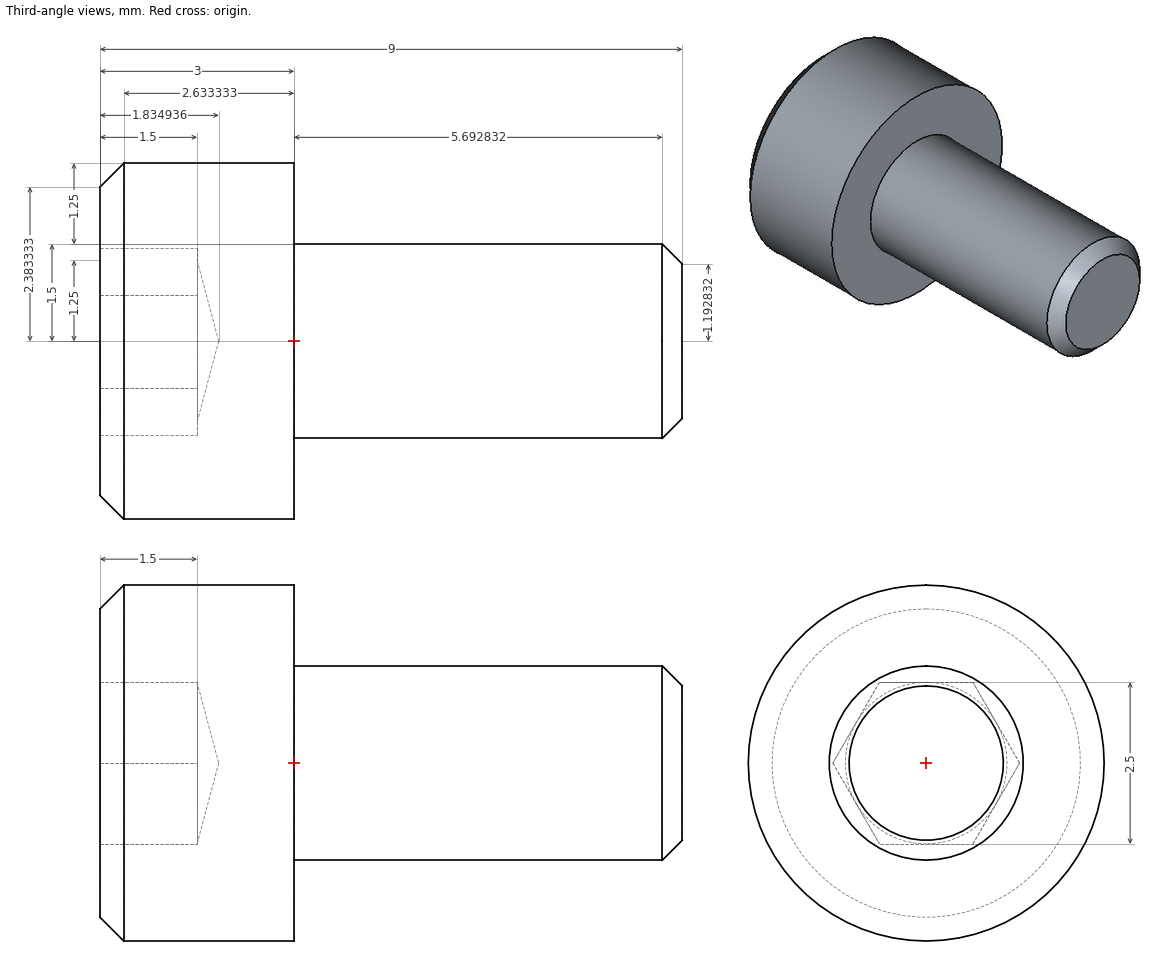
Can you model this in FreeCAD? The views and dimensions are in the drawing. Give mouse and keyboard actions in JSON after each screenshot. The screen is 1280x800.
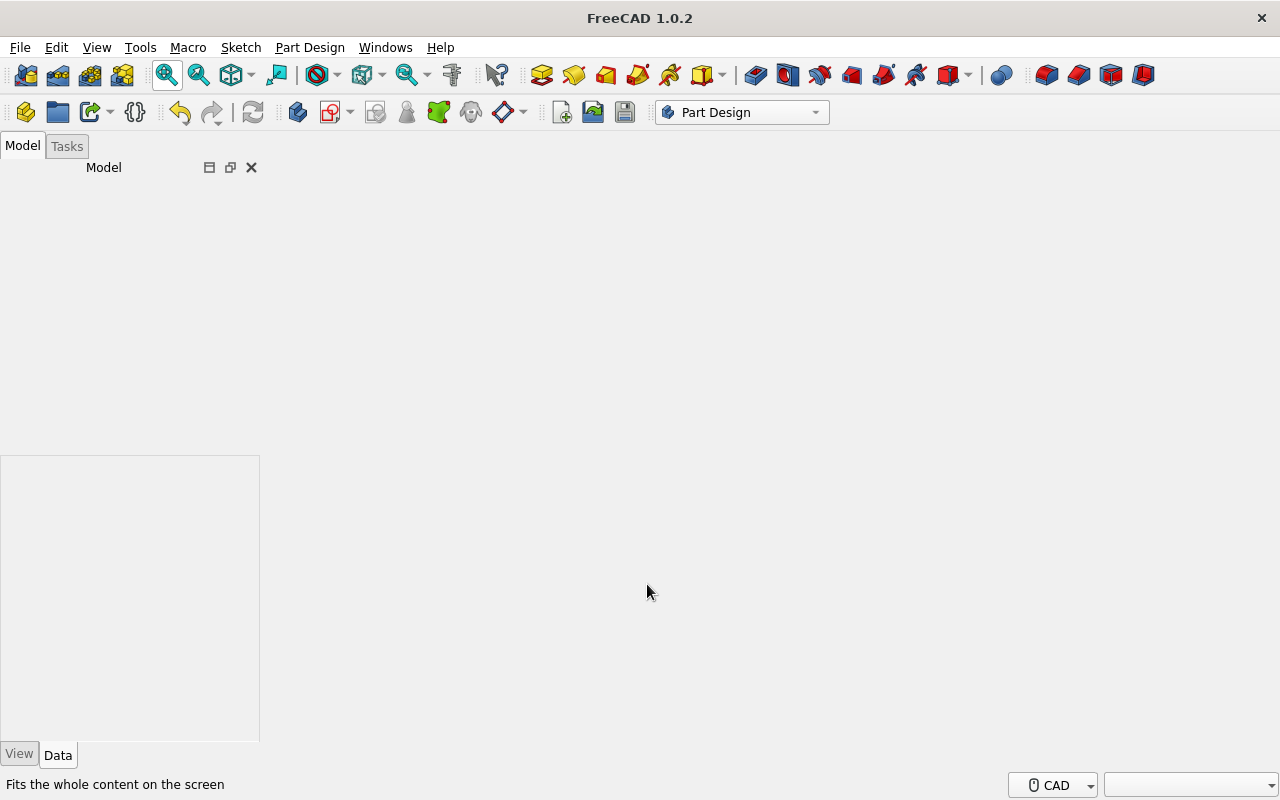
{"action": "left_click", "coordinate": [562, 112]}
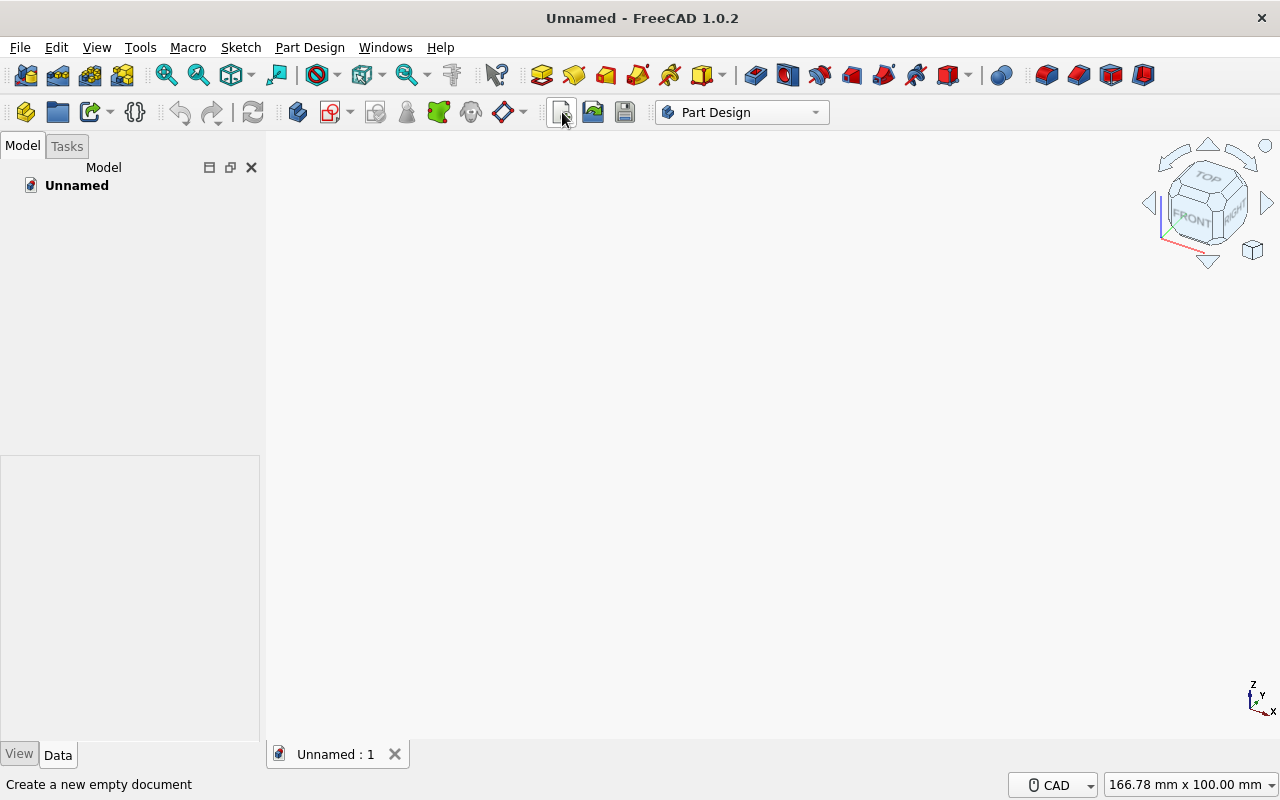
{"action": "left_click", "coordinate": [330, 112]}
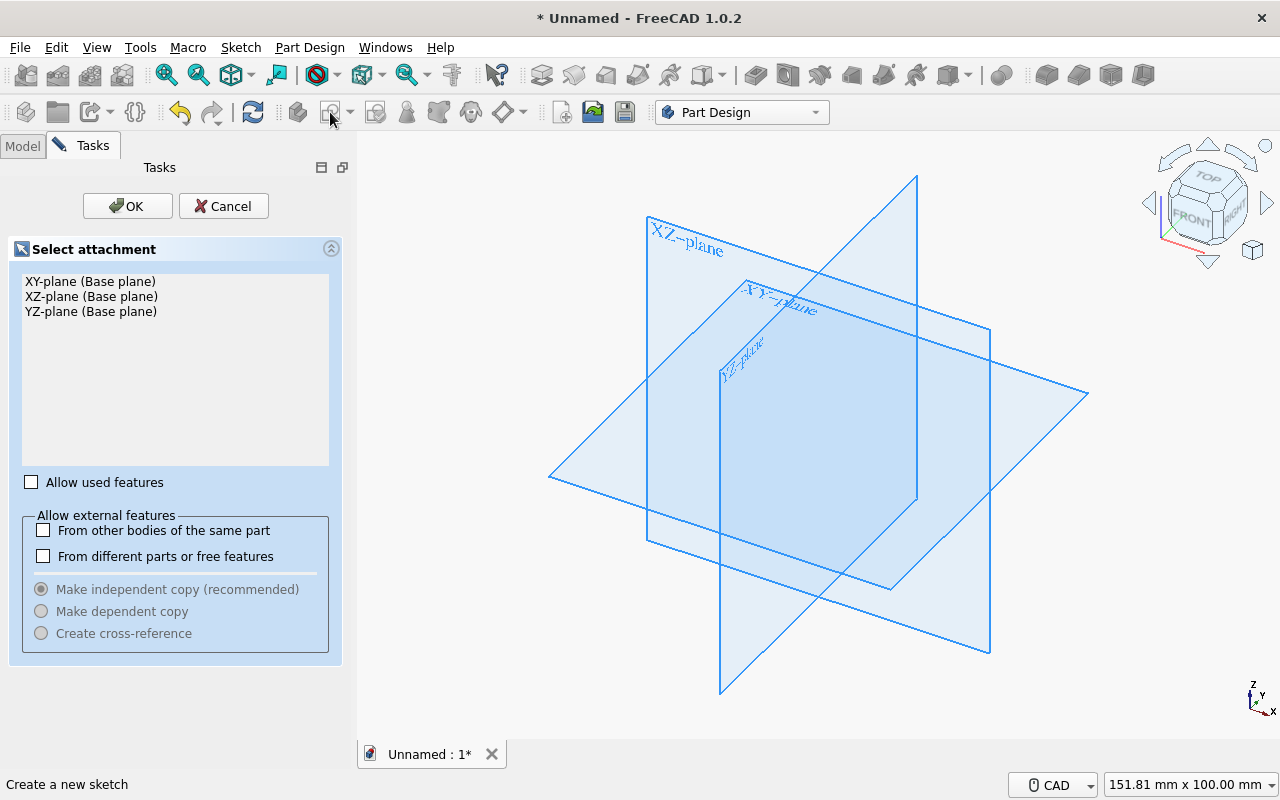
{"action": "left_click", "coordinate": [82, 282]}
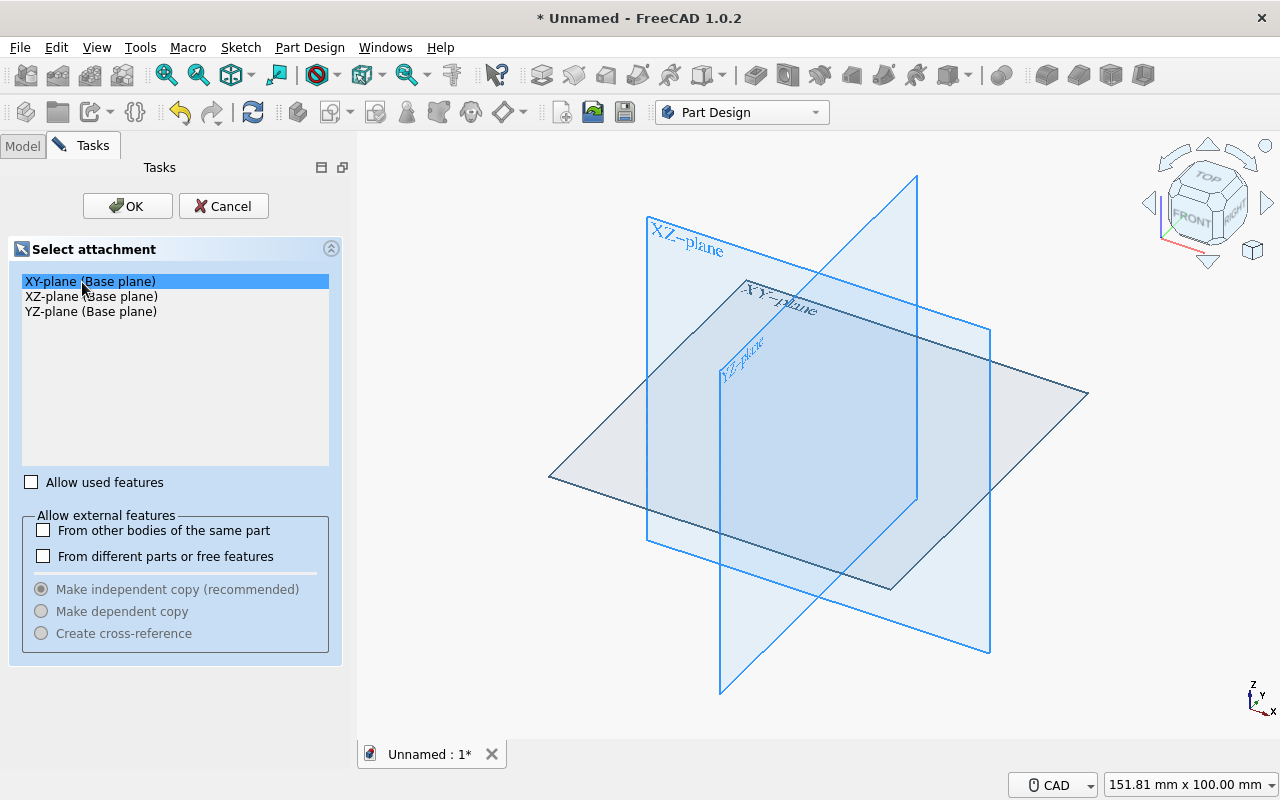
{"action": "left_click", "coordinate": [128, 206]}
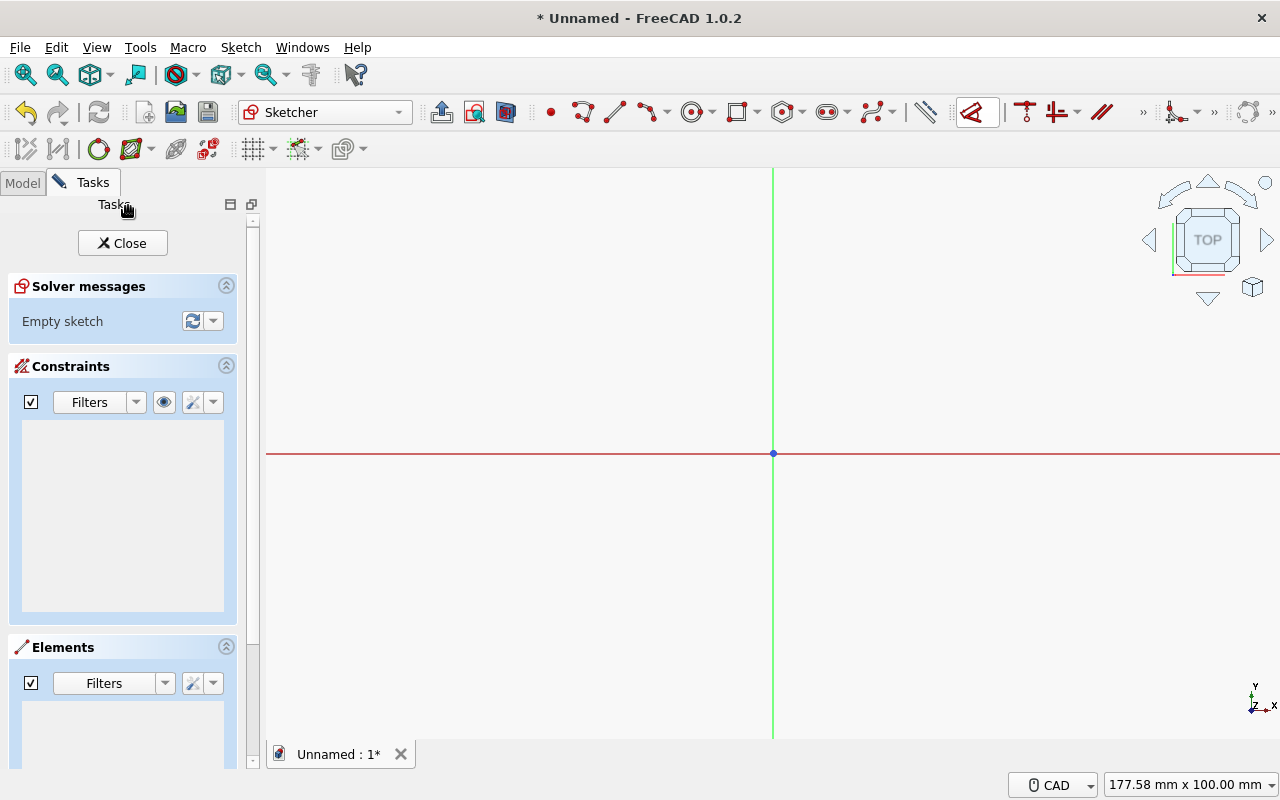
{"action": "scroll", "coordinate": [789, 445], "scroll_direction": "up", "scroll_amount": 12}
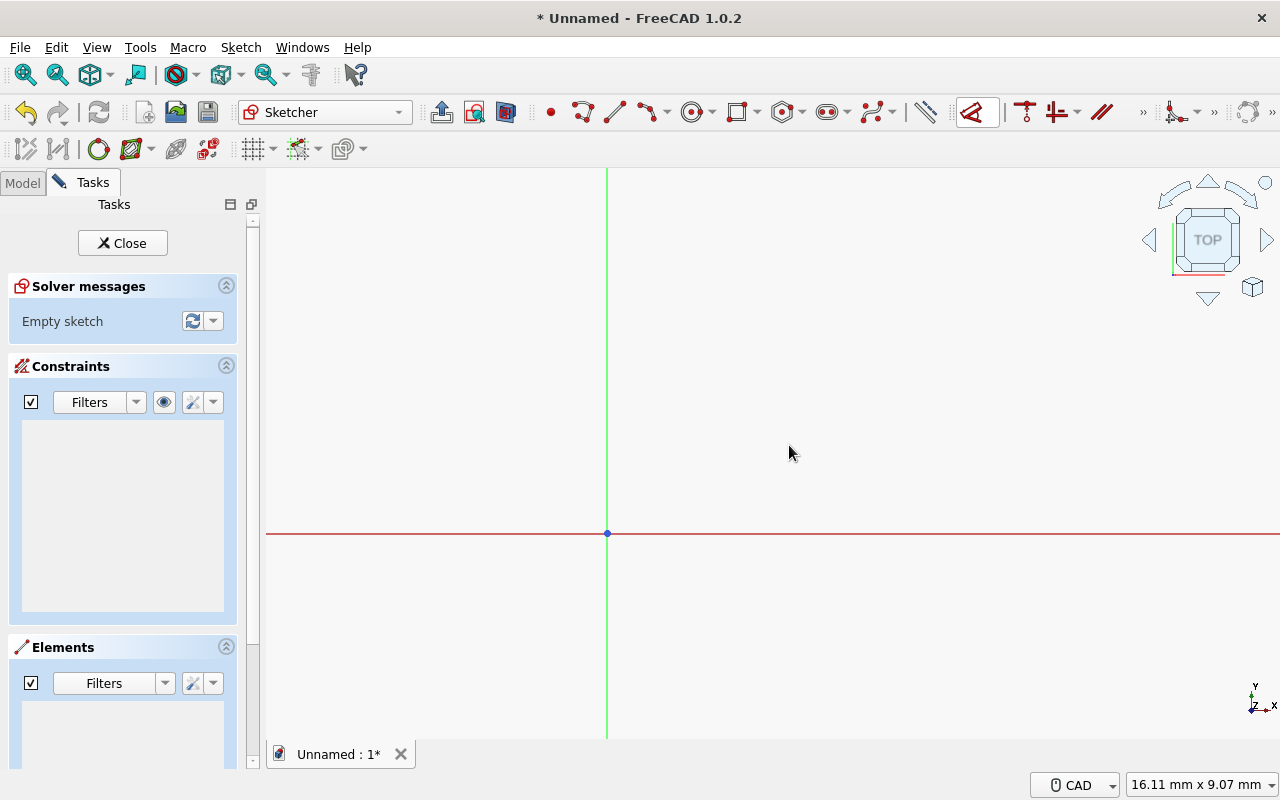
{"action": "left_click", "coordinate": [584, 112]}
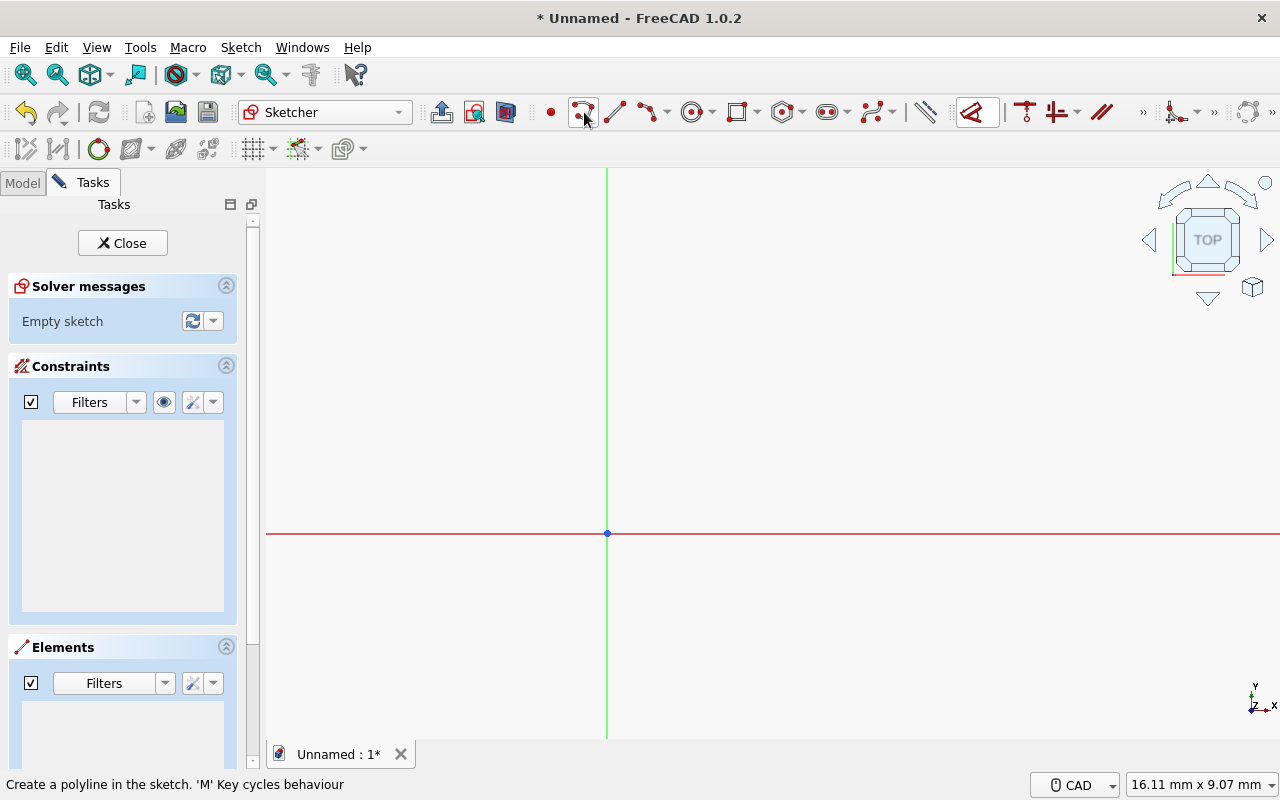
{"action": "left_click", "coordinate": [607, 439]}
{"action": "left_click", "coordinate": [616, 361]}
{"action": "left_click", "coordinate": [442, 361]}
{"action": "left_click", "coordinate": [419, 384]}
{"action": "left_click", "coordinate": [419, 534]}
{"action": "left_click", "coordinate": [985, 525]}
{"action": "left_click", "coordinate": [985, 459]}
{"action": "left_click", "coordinate": [966, 439]}
{"action": "left_click", "coordinate": [607, 440]}
{"action": "key", "text": "Escape"}
{"action": "key", "text": "Escape"}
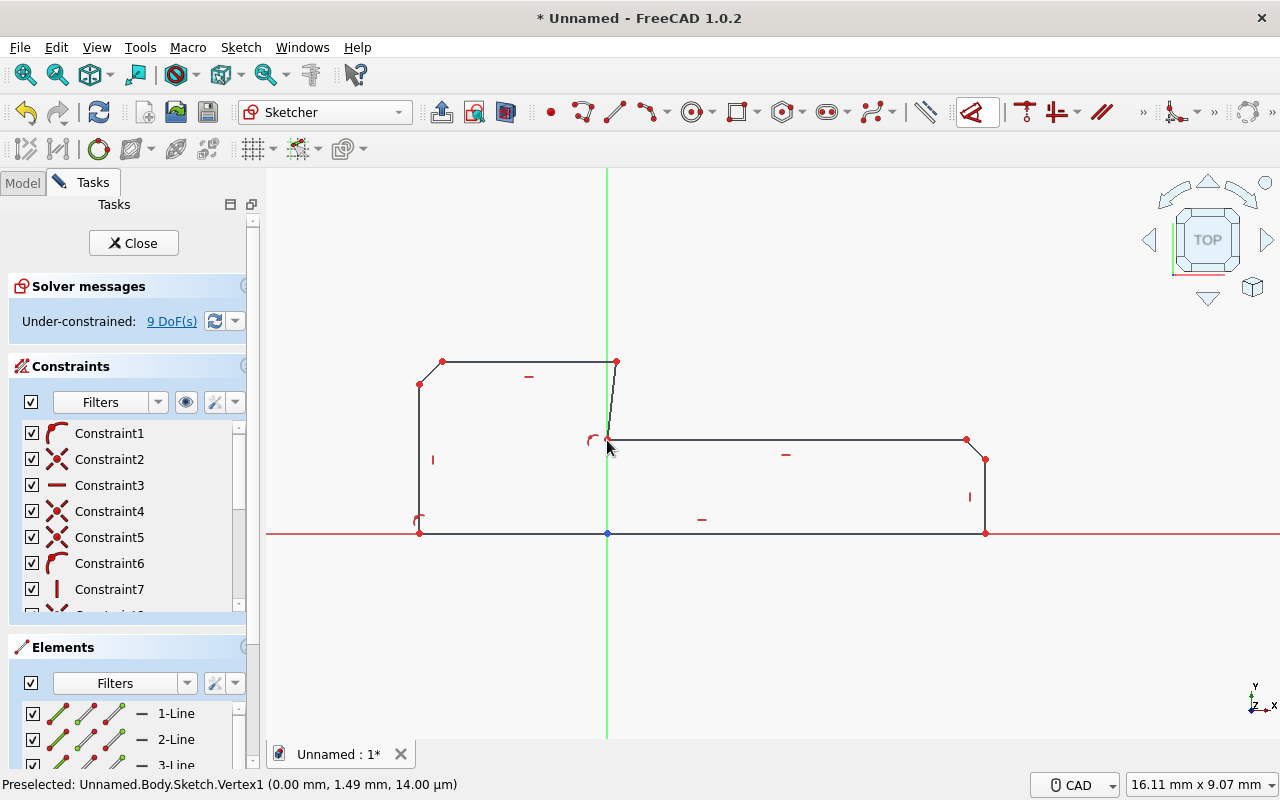
{"action": "left_click", "coordinate": [610, 417]}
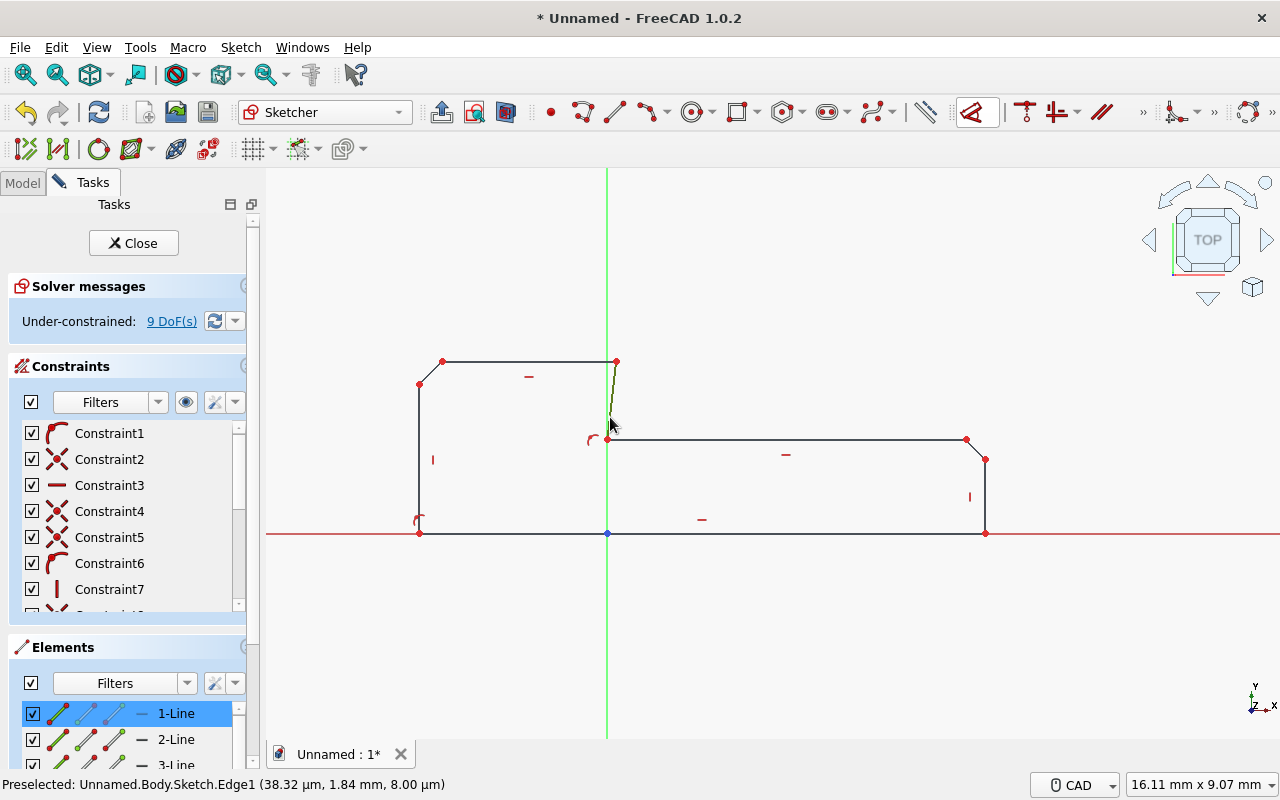
{"action": "key", "text": "v"}